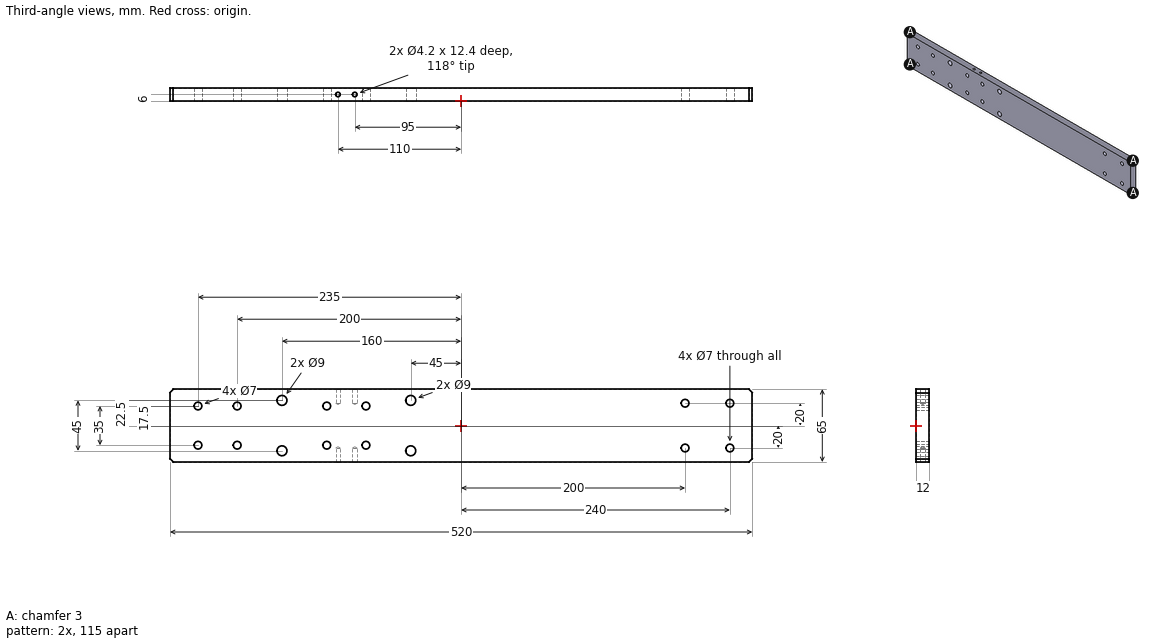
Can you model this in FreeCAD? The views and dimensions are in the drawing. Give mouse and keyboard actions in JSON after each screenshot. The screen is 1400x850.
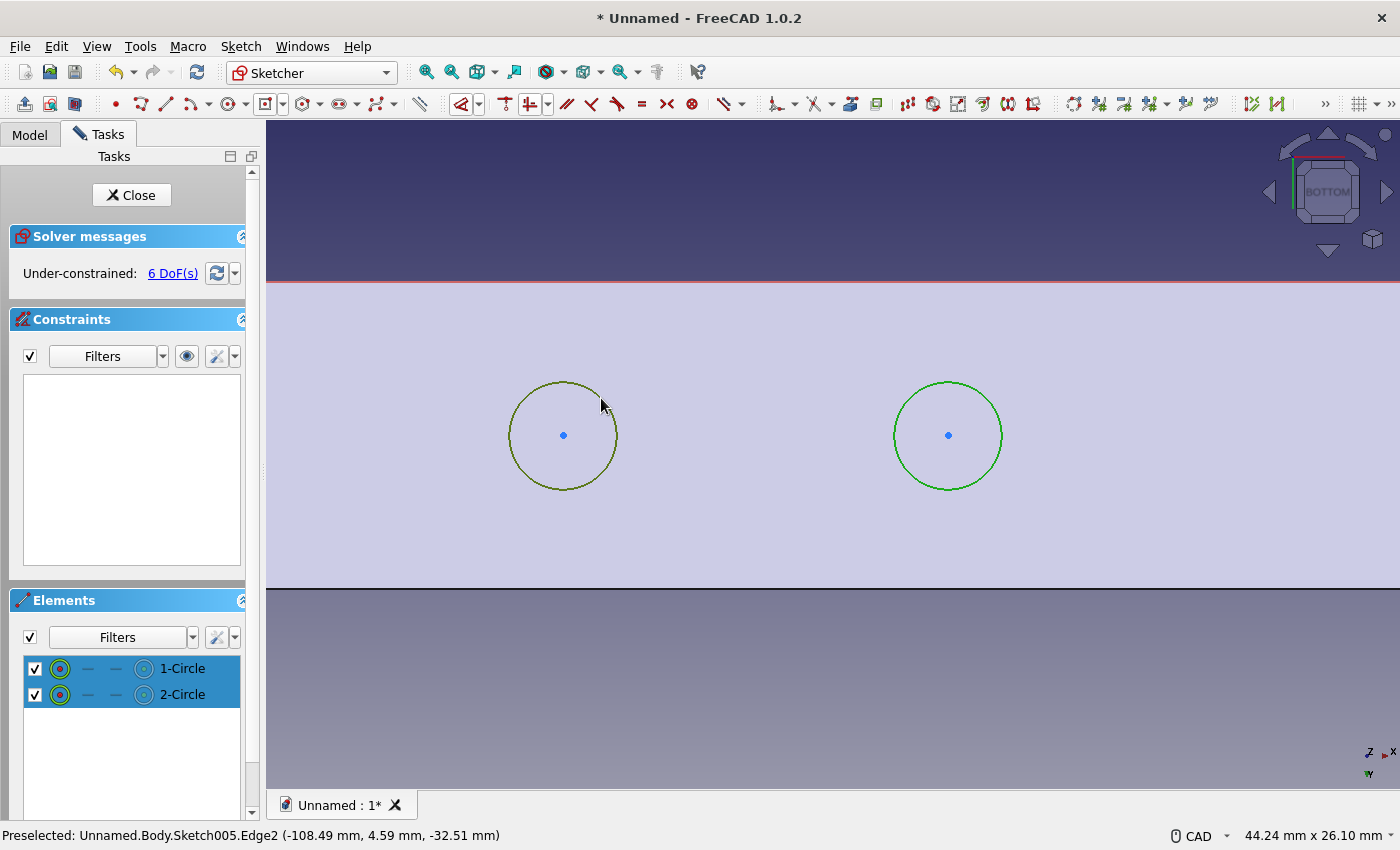
{"action": "left_click", "coordinate": [642, 104]}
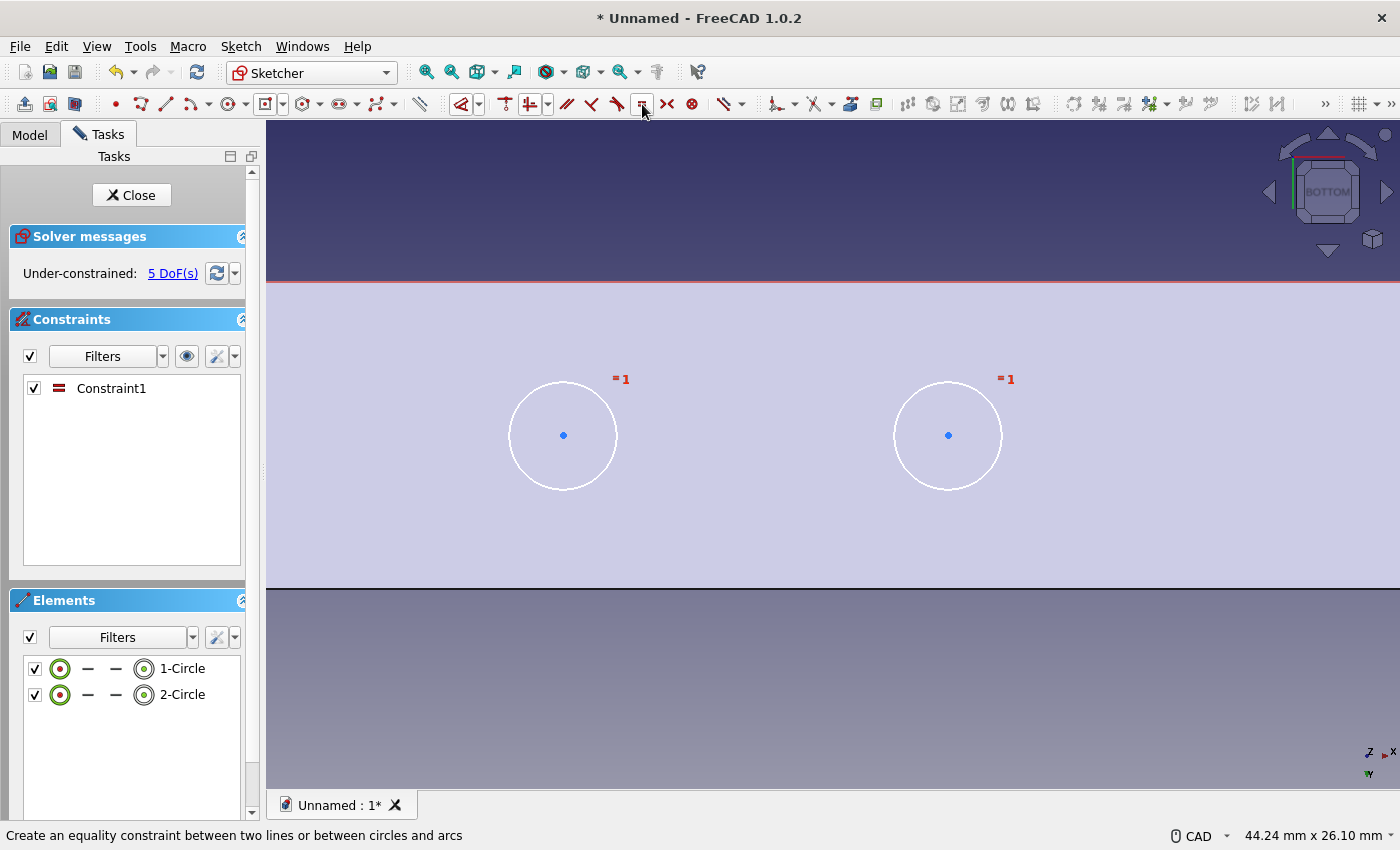
{"action": "left_click", "coordinate": [948, 436]}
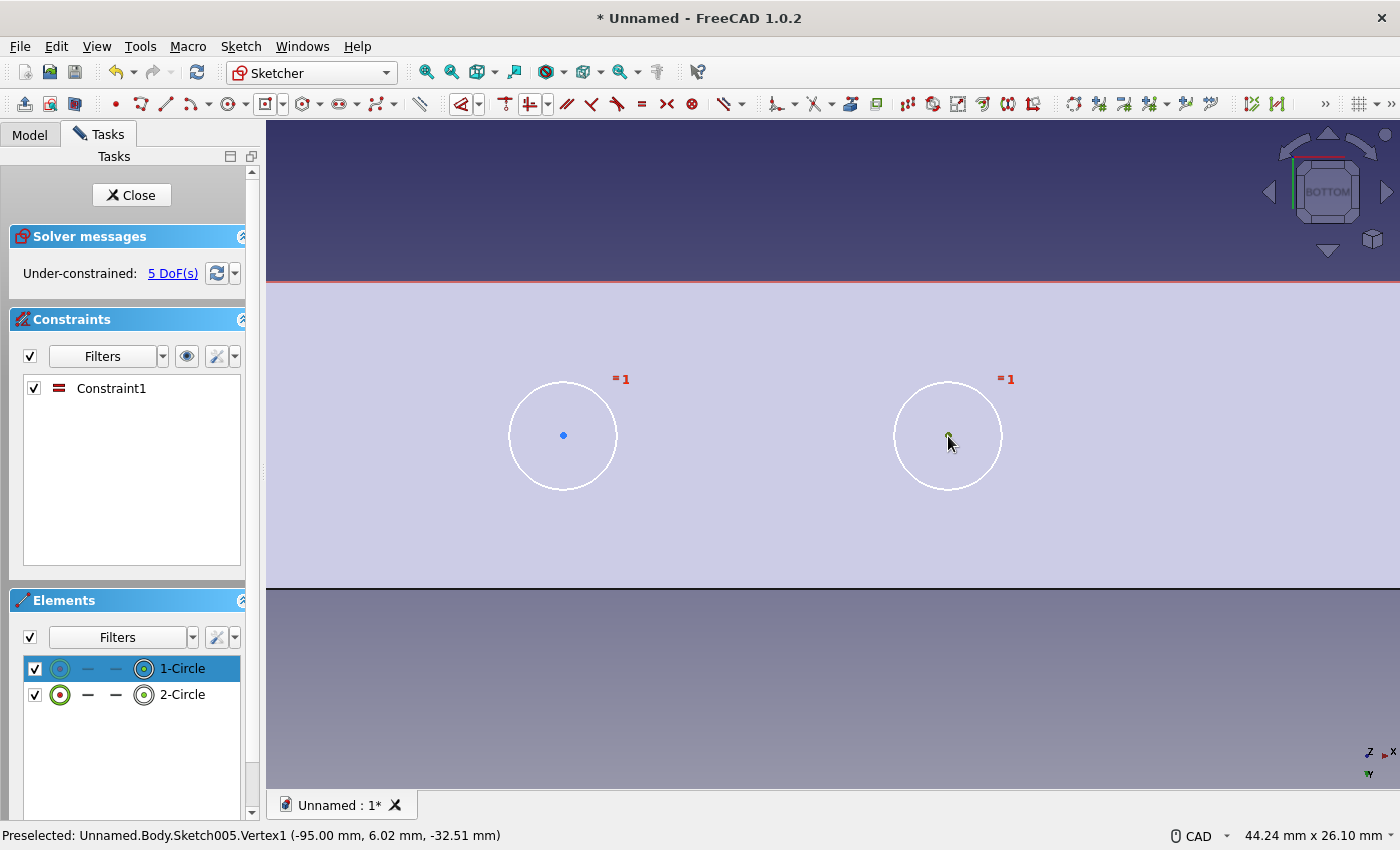
{"action": "left_click", "coordinate": [563, 436]}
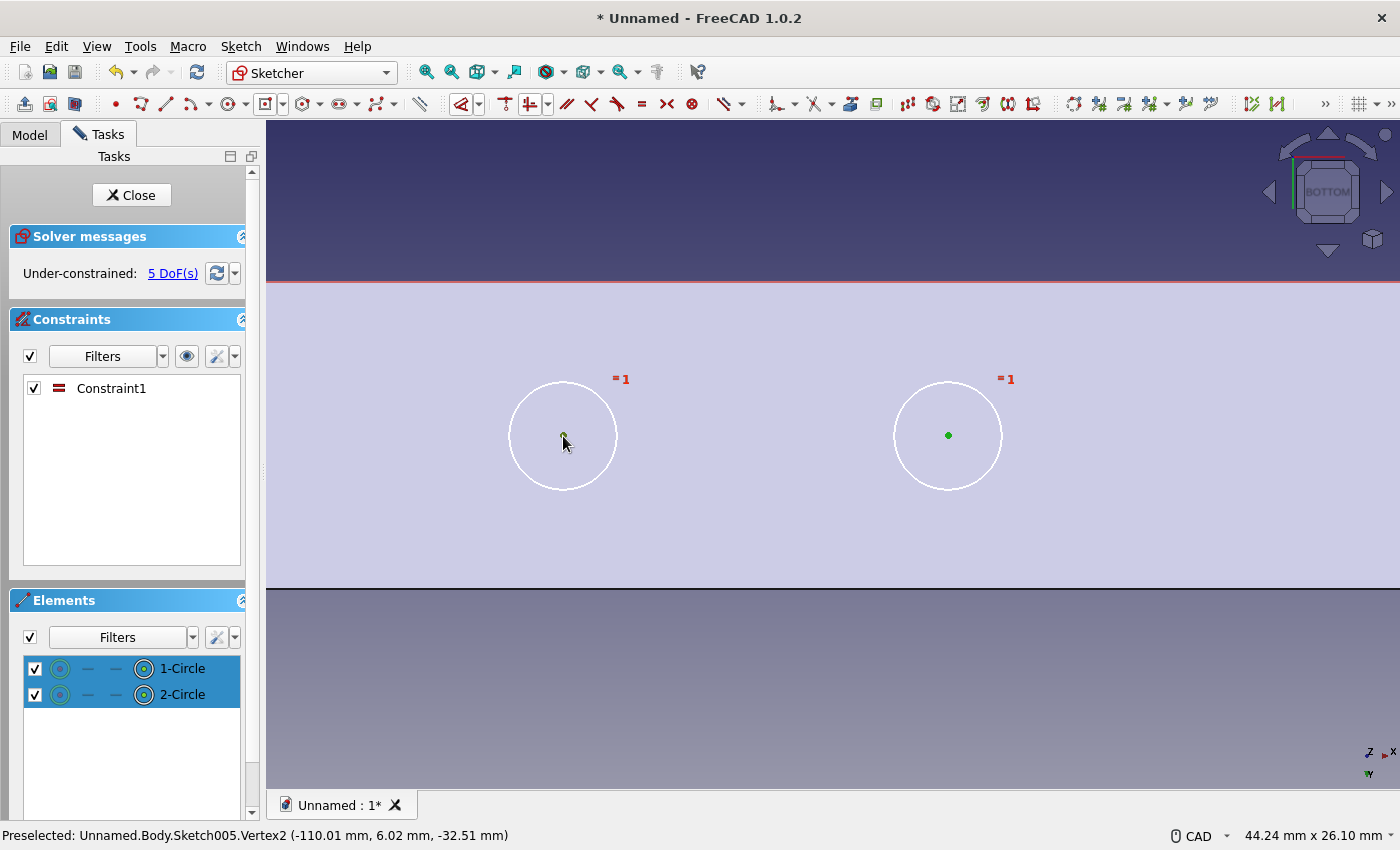
{"action": "key", "text": "h"}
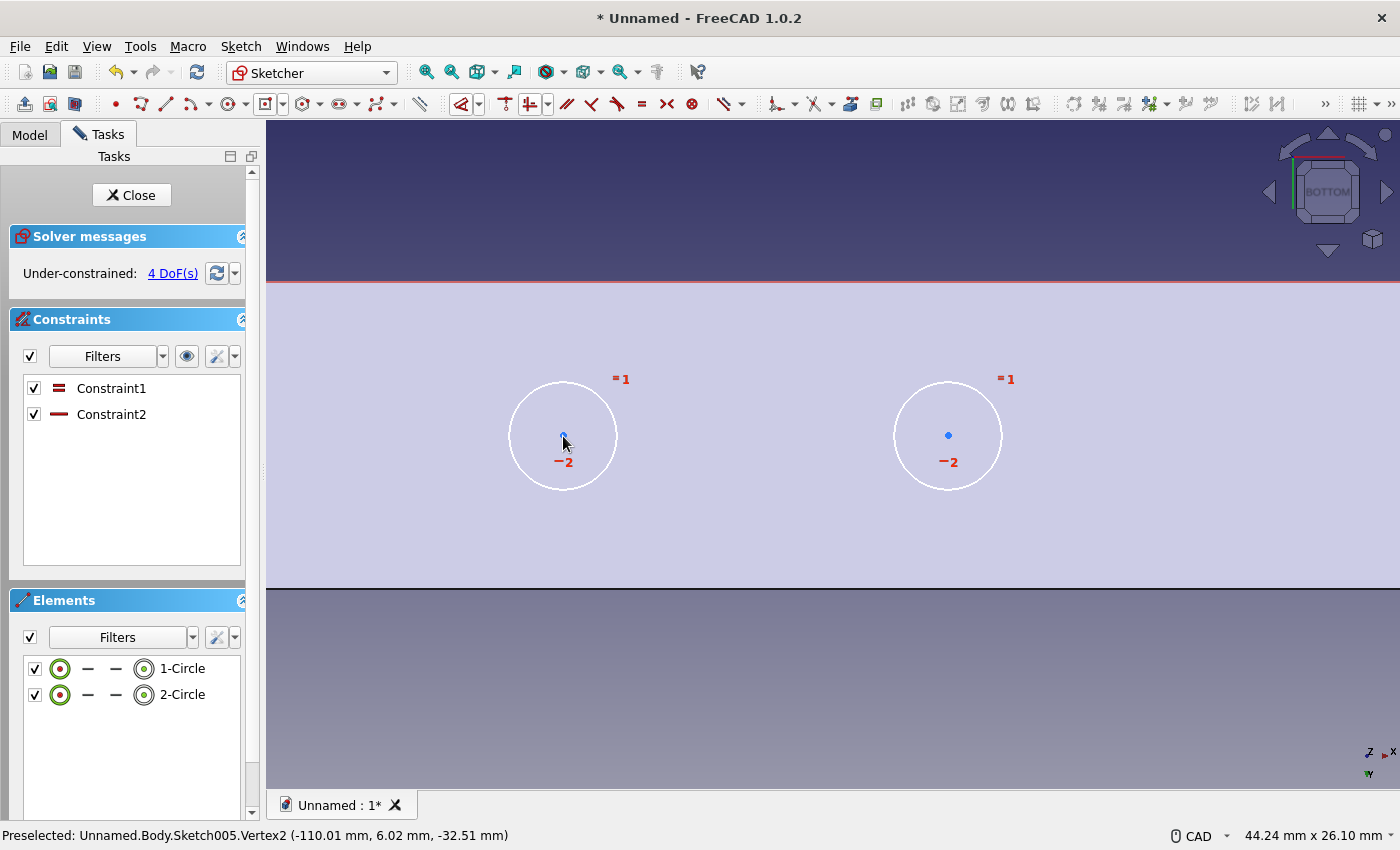
{"action": "left_click", "coordinate": [986, 398]}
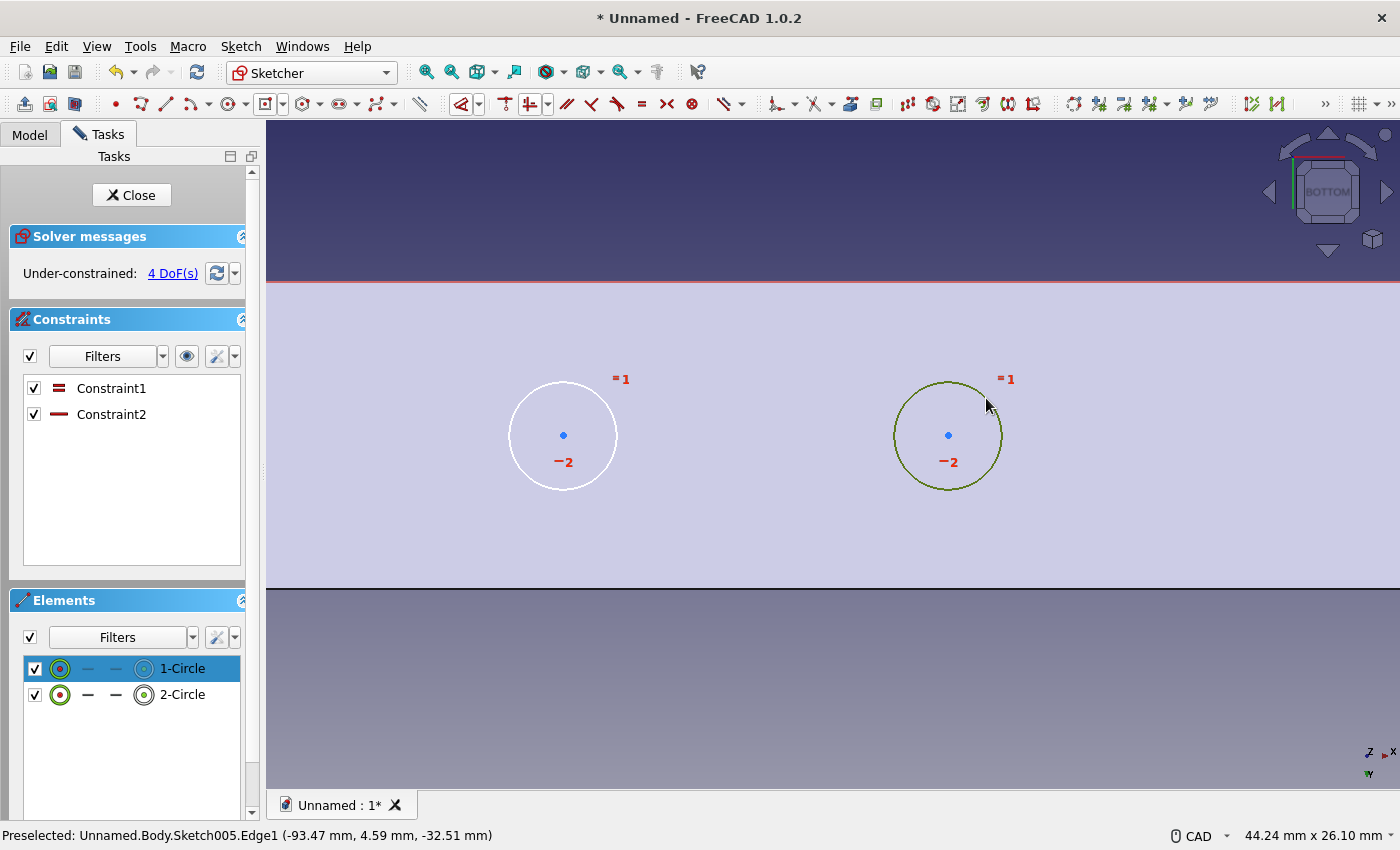
{"action": "key", "text": "k o"}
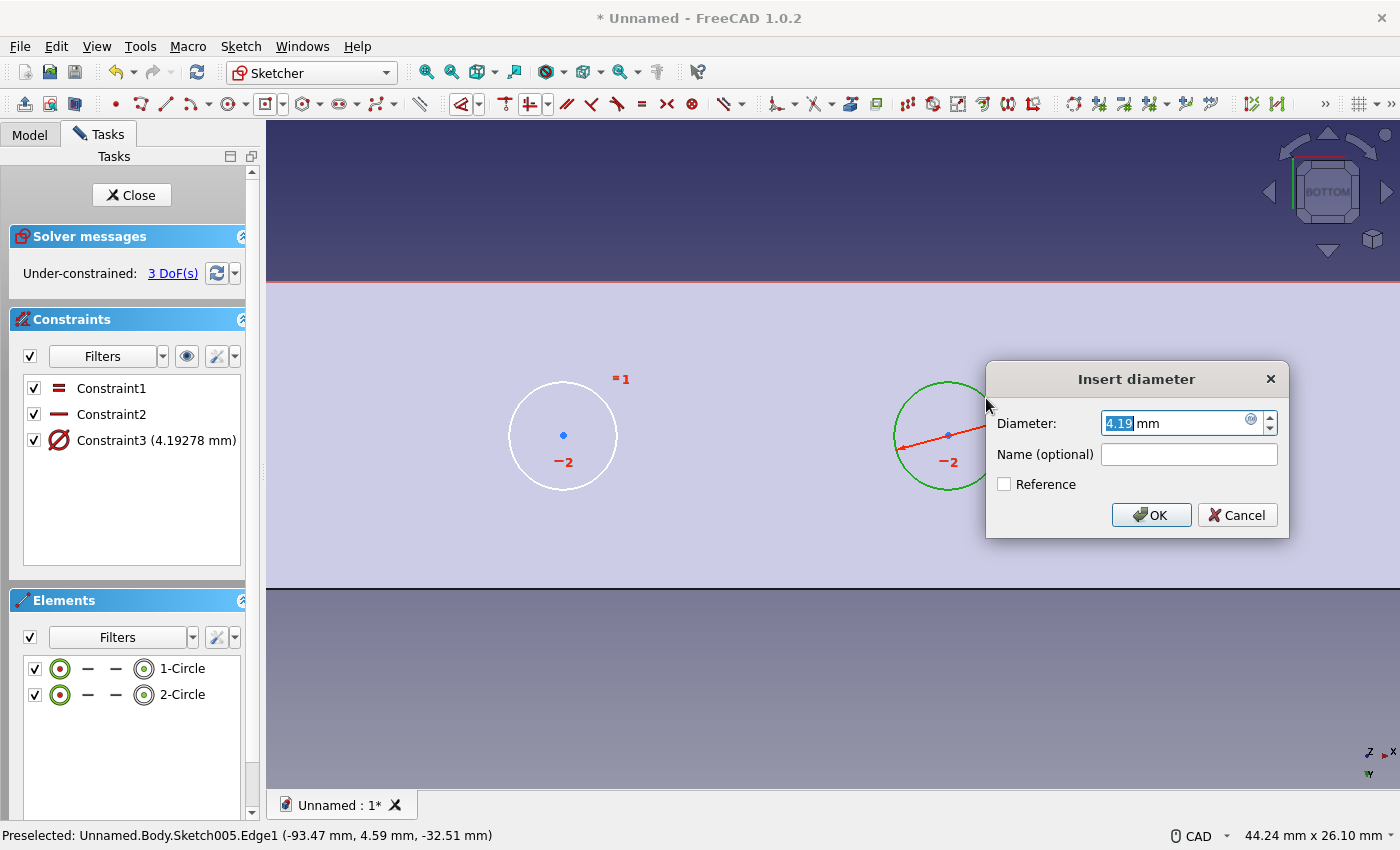
{"action": "type", "text": "4.2"}
{"action": "key", "text": "Return"}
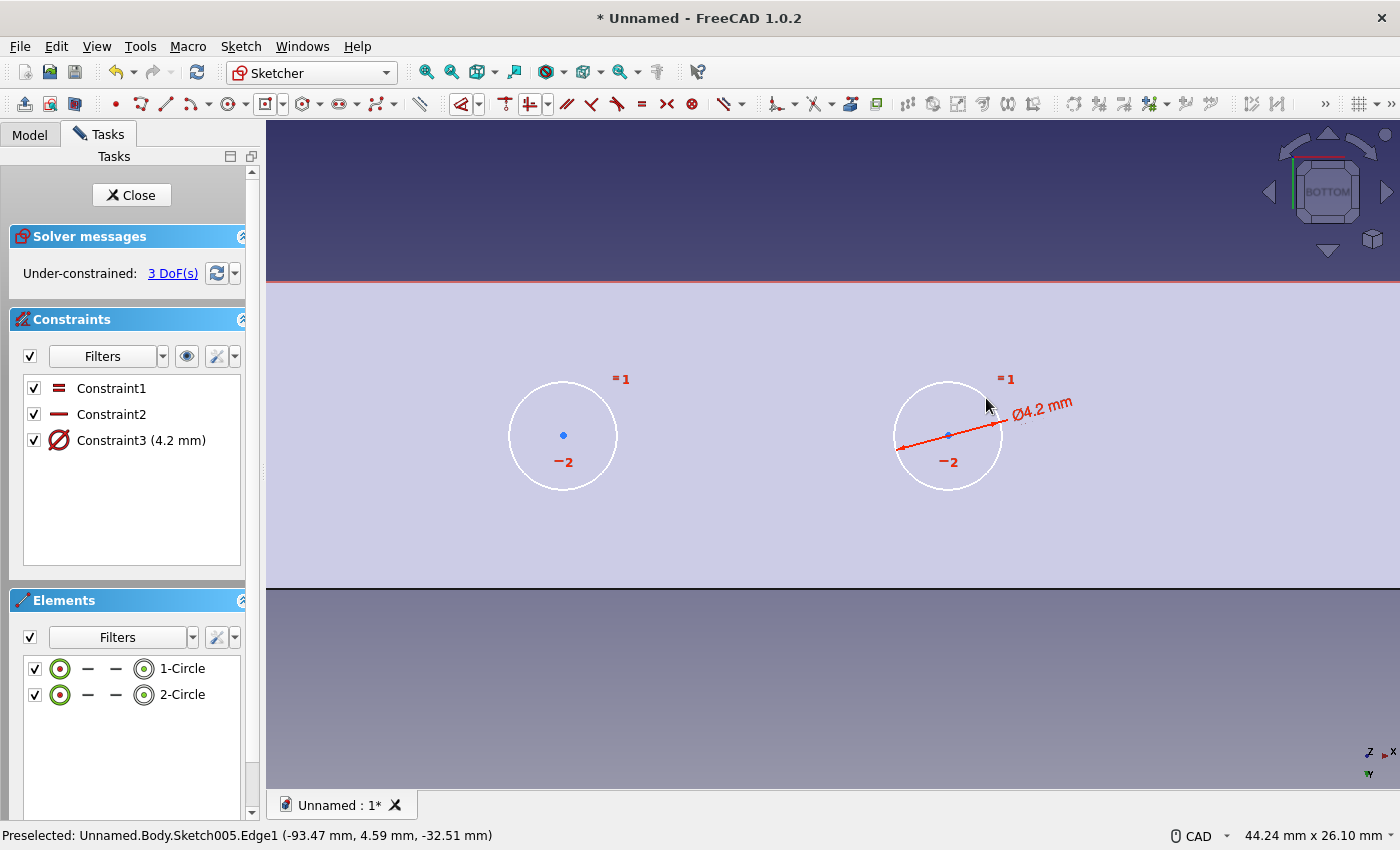
{"action": "left_click", "coordinate": [948, 436]}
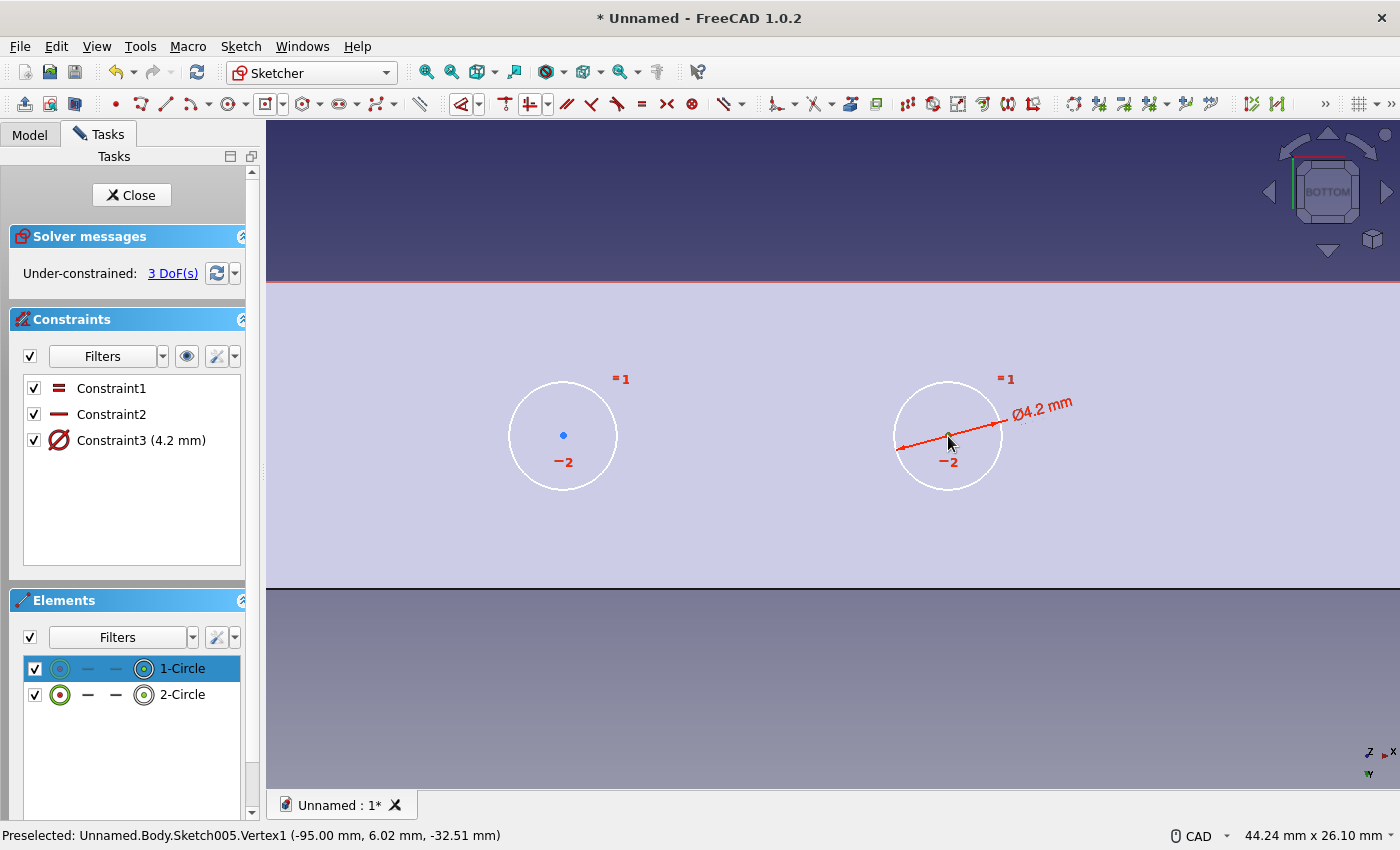
{"action": "left_click", "coordinate": [478, 104]}